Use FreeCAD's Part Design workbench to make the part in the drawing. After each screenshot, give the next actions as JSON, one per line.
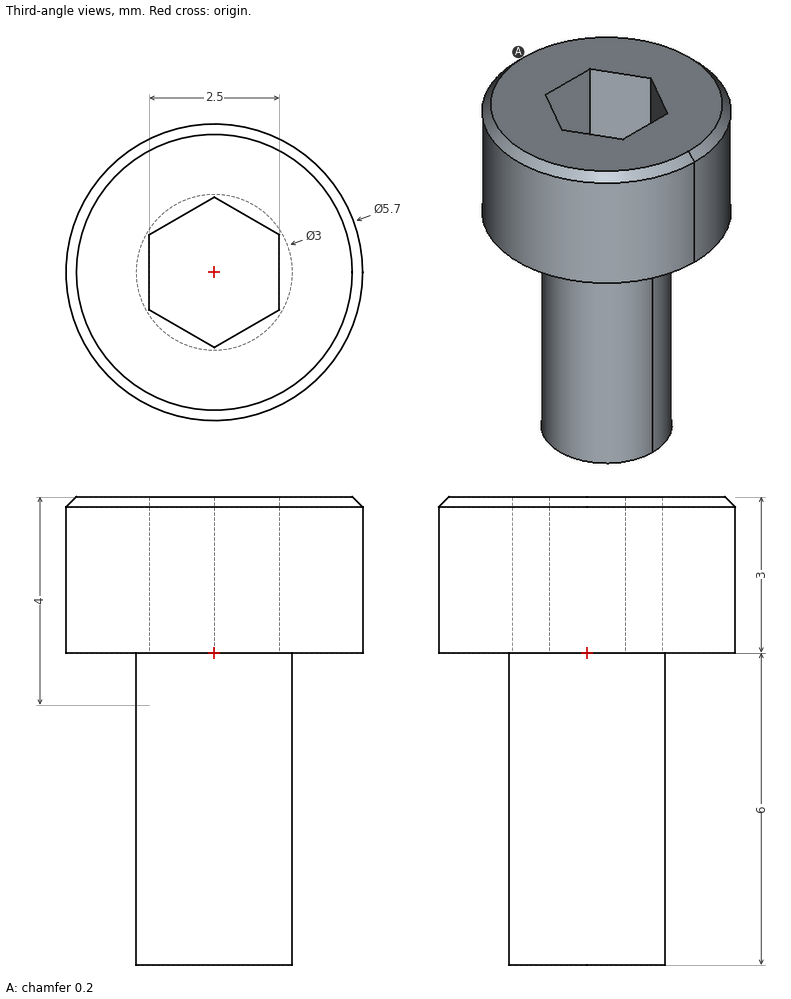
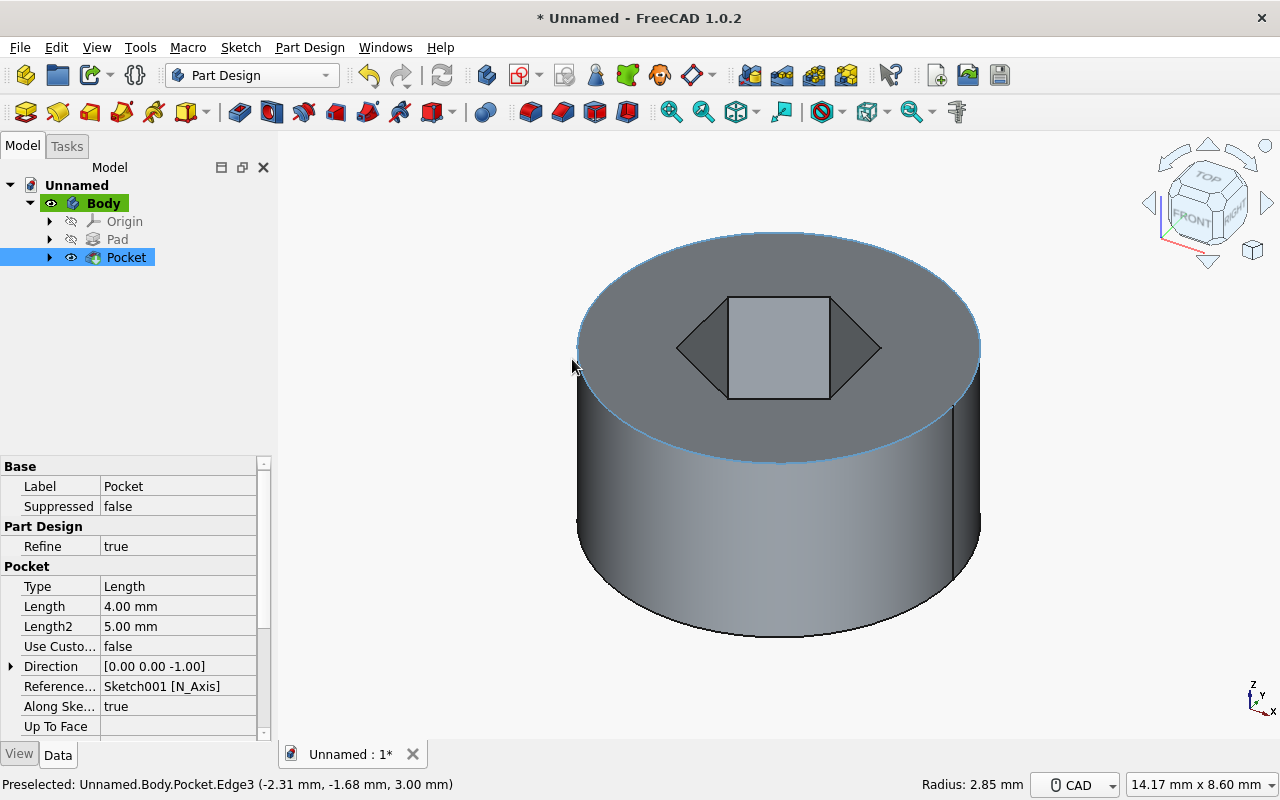
{"action": "left_click", "coordinate": [564, 112]}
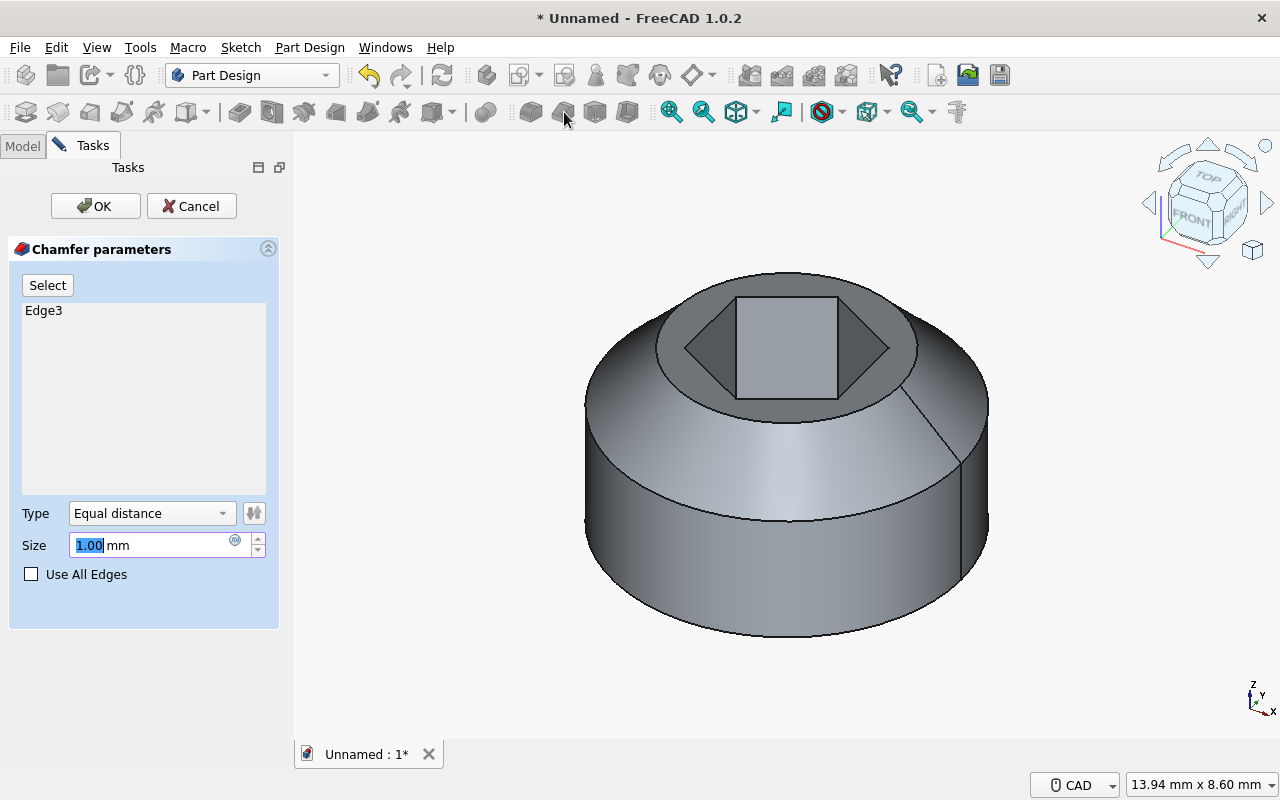
{"action": "type", "text": "0.2"}
{"action": "key", "text": "Tab"}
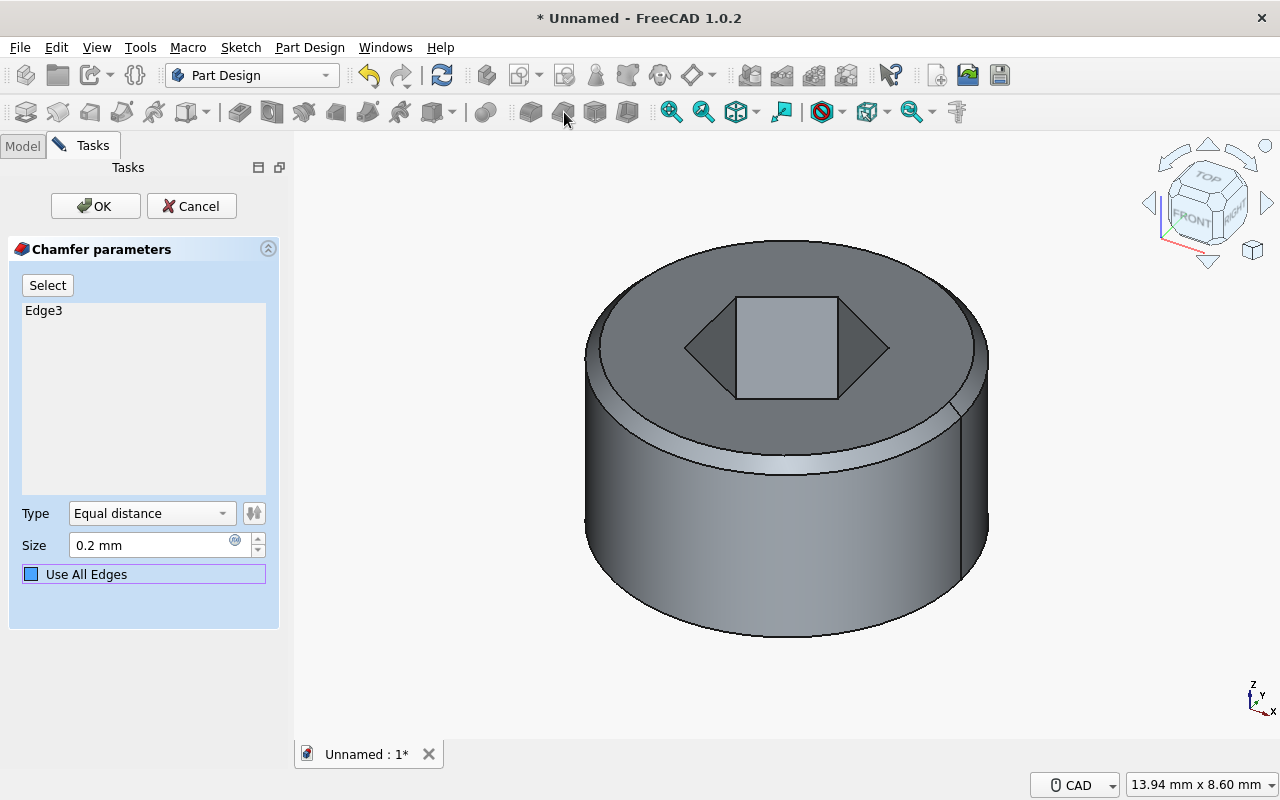
{"action": "left_click", "coordinate": [96, 206]}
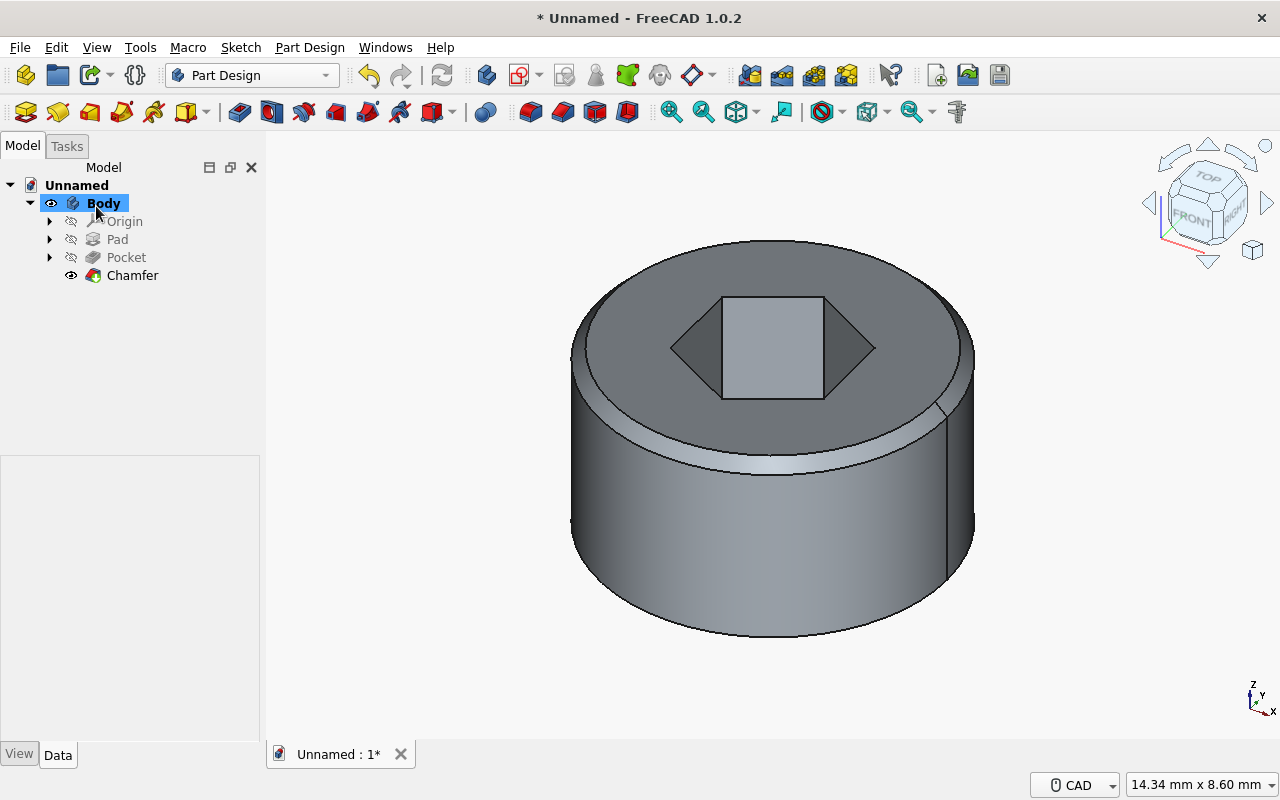
{"action": "left_click", "coordinate": [520, 76]}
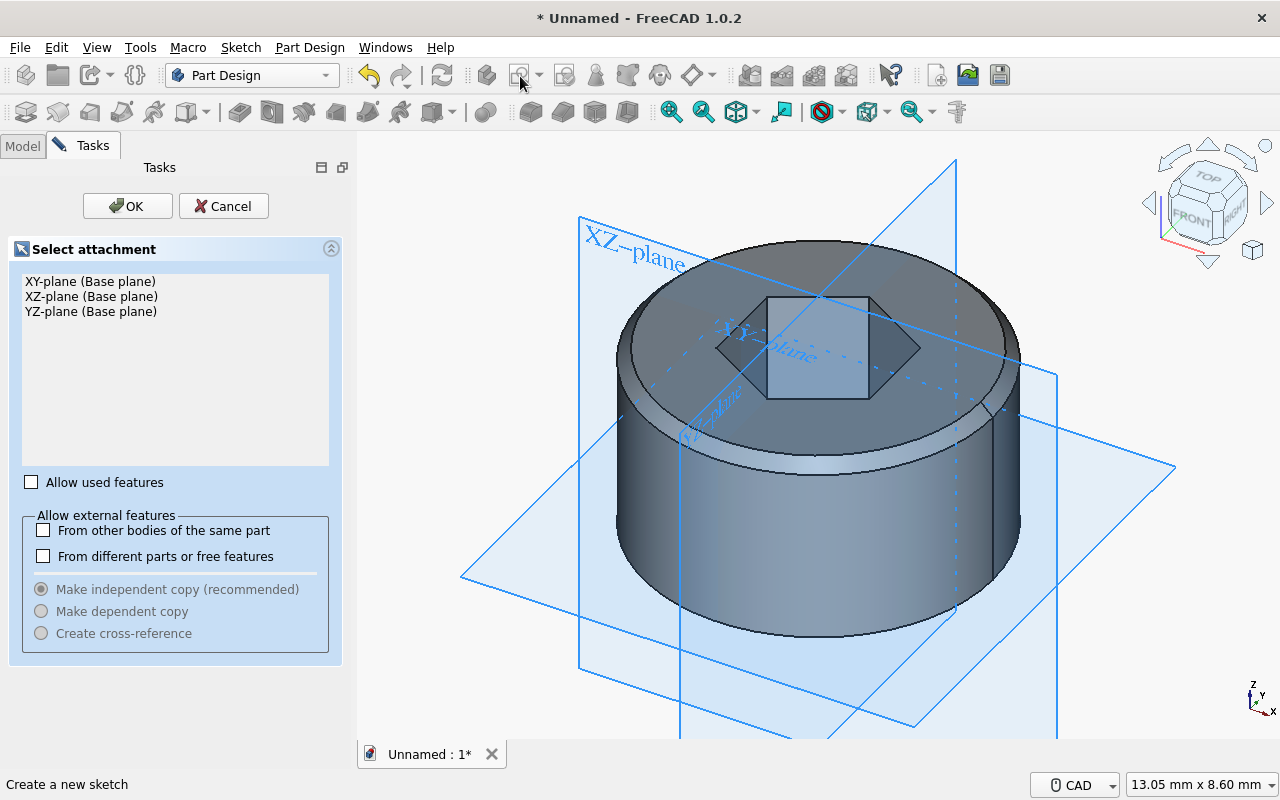
{"action": "left_click", "coordinate": [82, 282]}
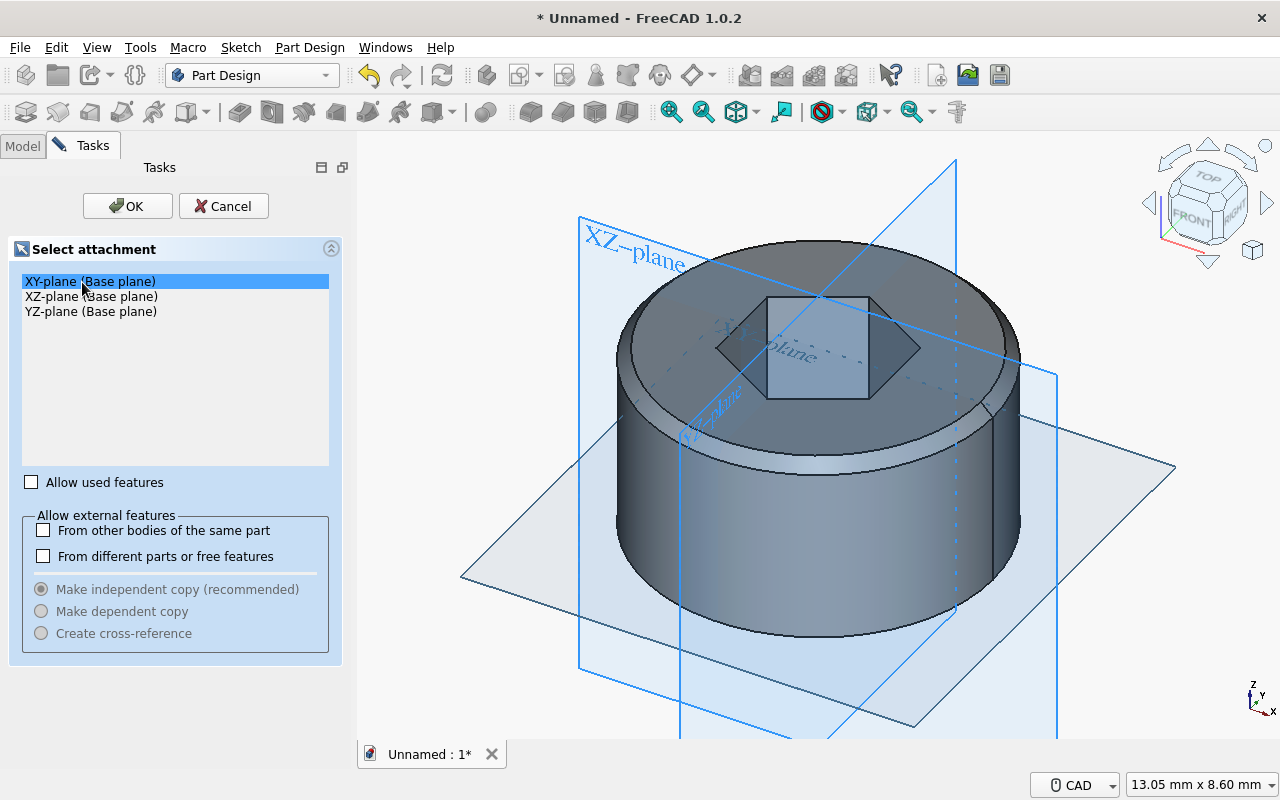
{"action": "left_click", "coordinate": [128, 206]}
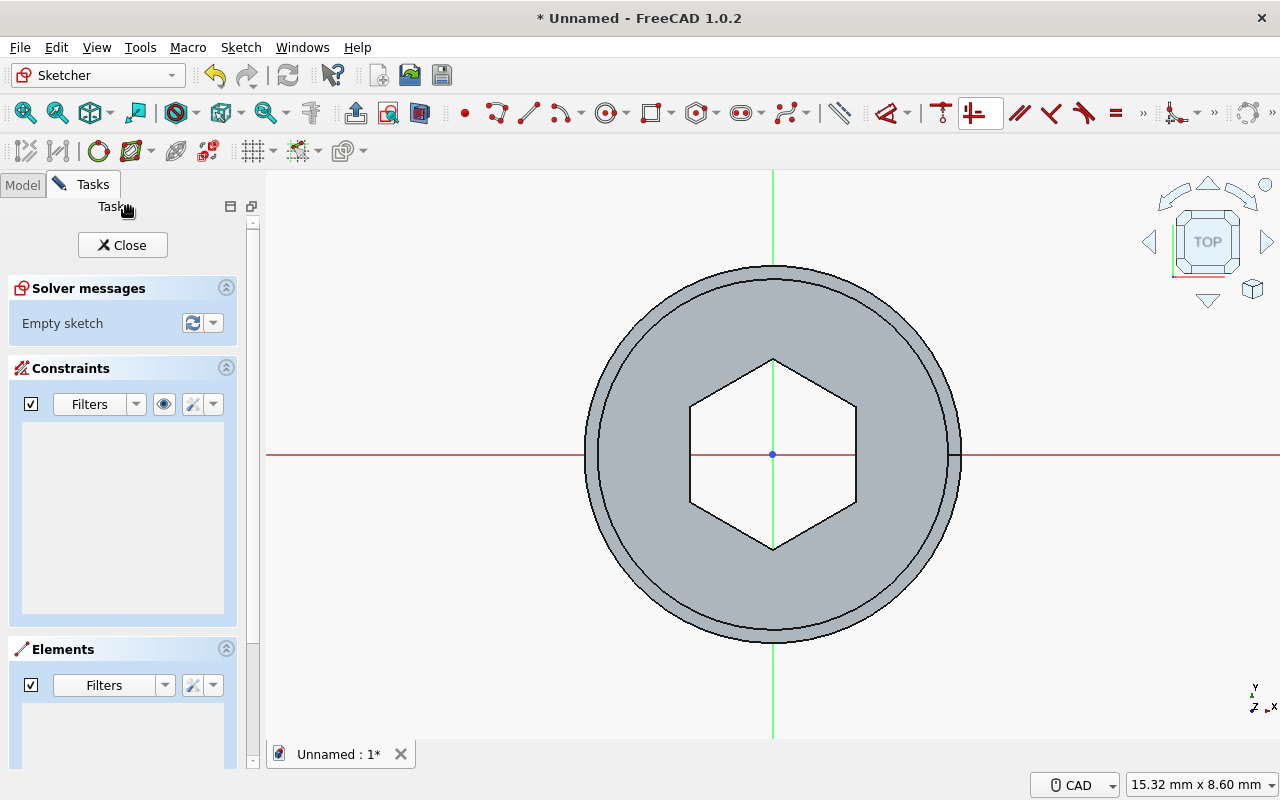
{"action": "left_click", "coordinate": [420, 114]}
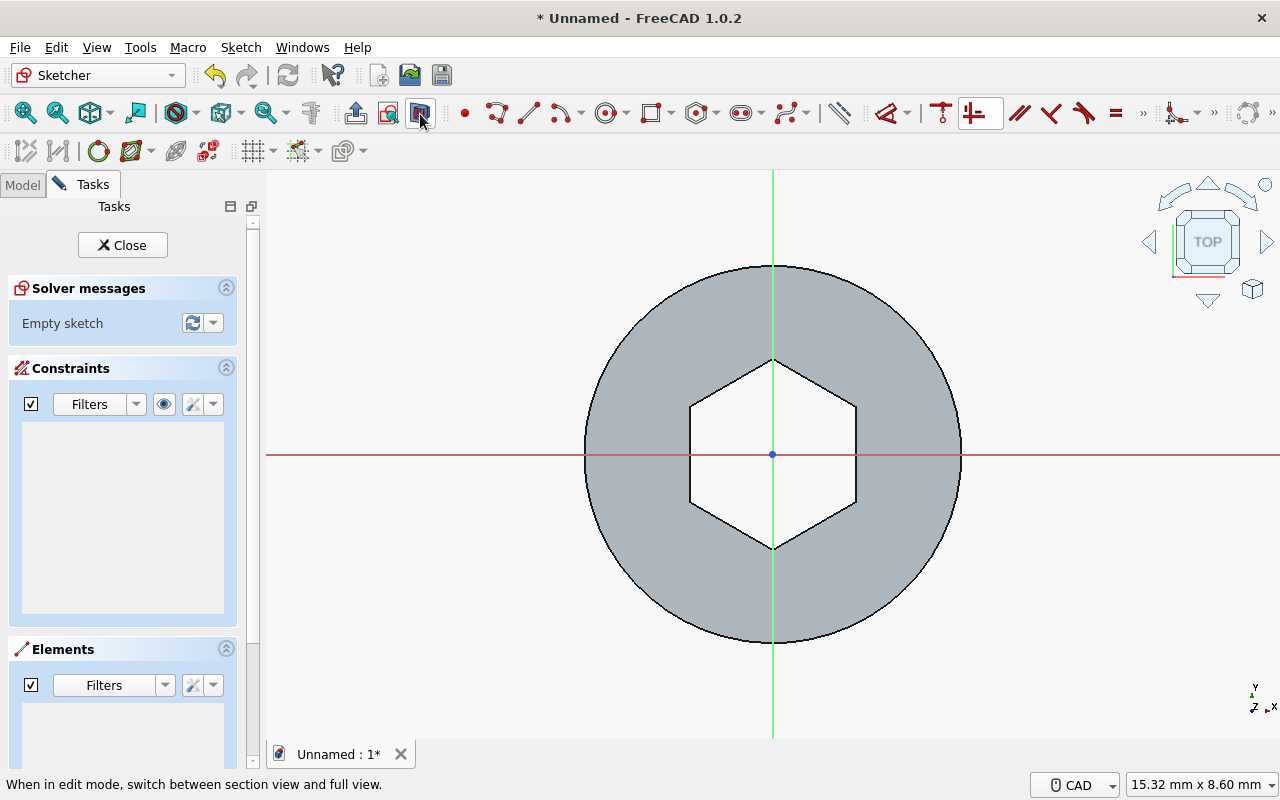
{"action": "scroll", "coordinate": [856, 454], "scroll_direction": "up", "scroll_amount": 3}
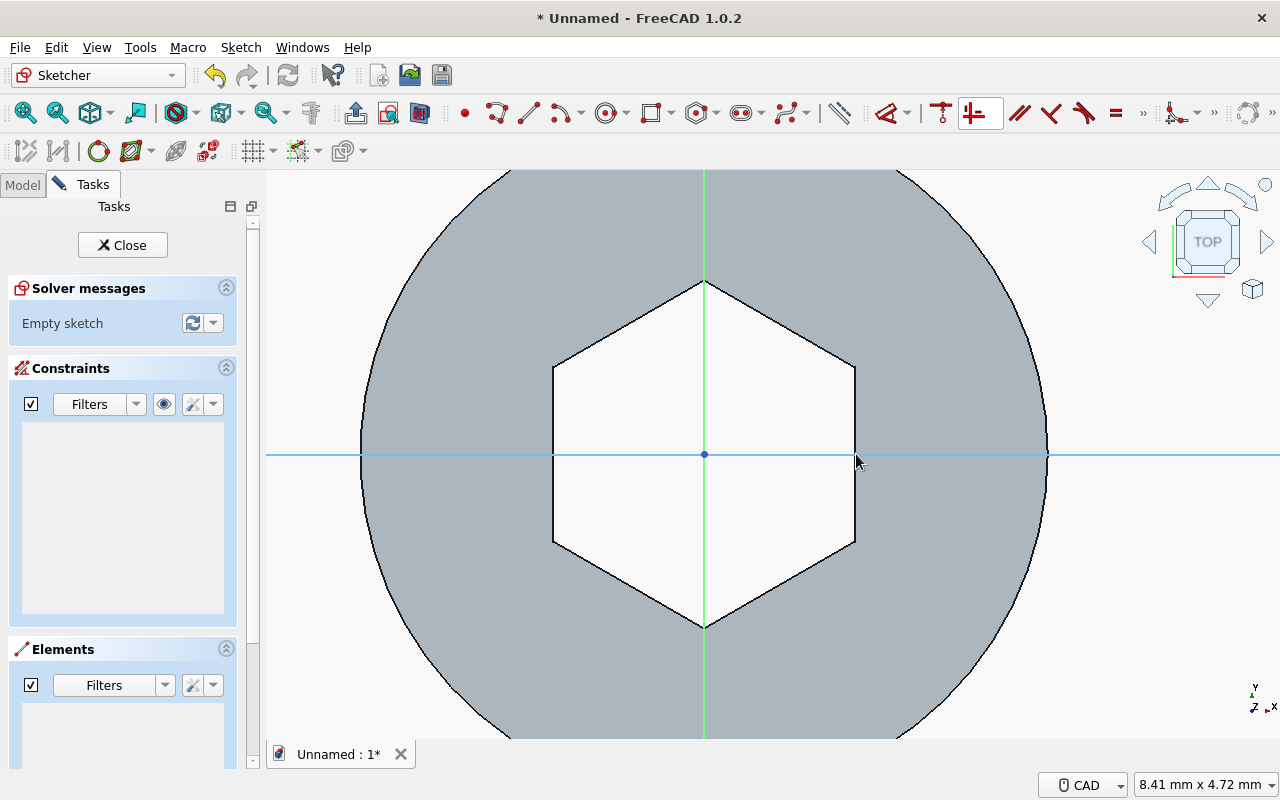
{"action": "key", "text": "g c"}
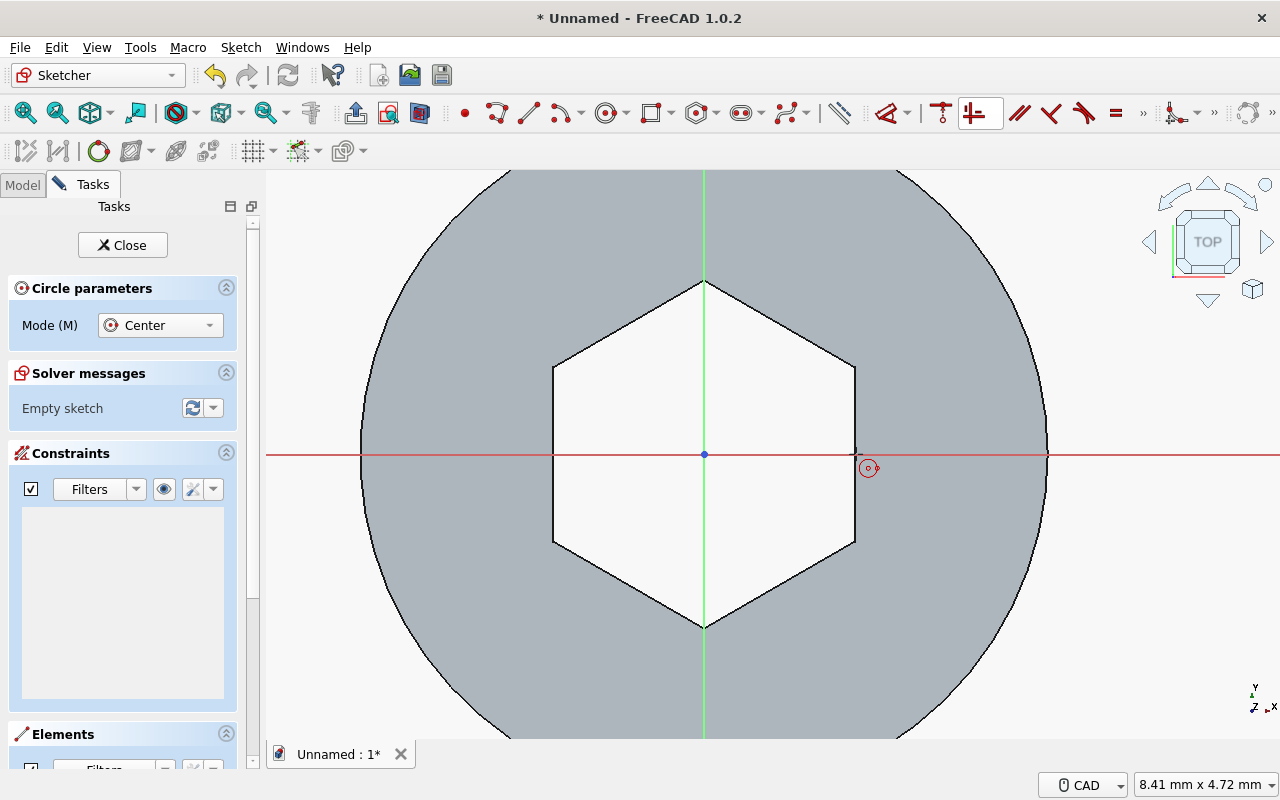
{"action": "left_click", "coordinate": [704, 454]}
{"action": "left_click", "coordinate": [832, 327]}
{"action": "key", "text": "Escape"}